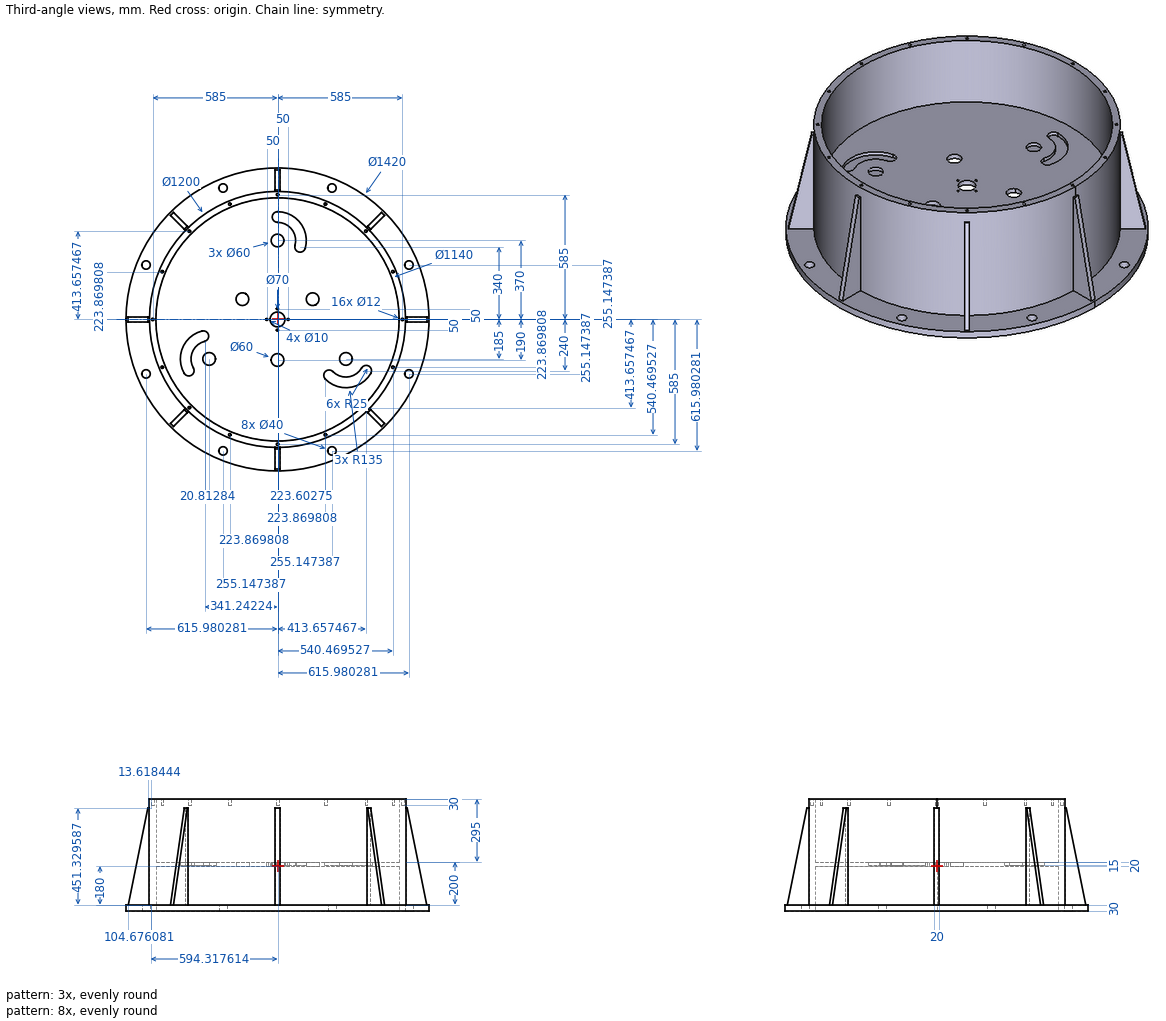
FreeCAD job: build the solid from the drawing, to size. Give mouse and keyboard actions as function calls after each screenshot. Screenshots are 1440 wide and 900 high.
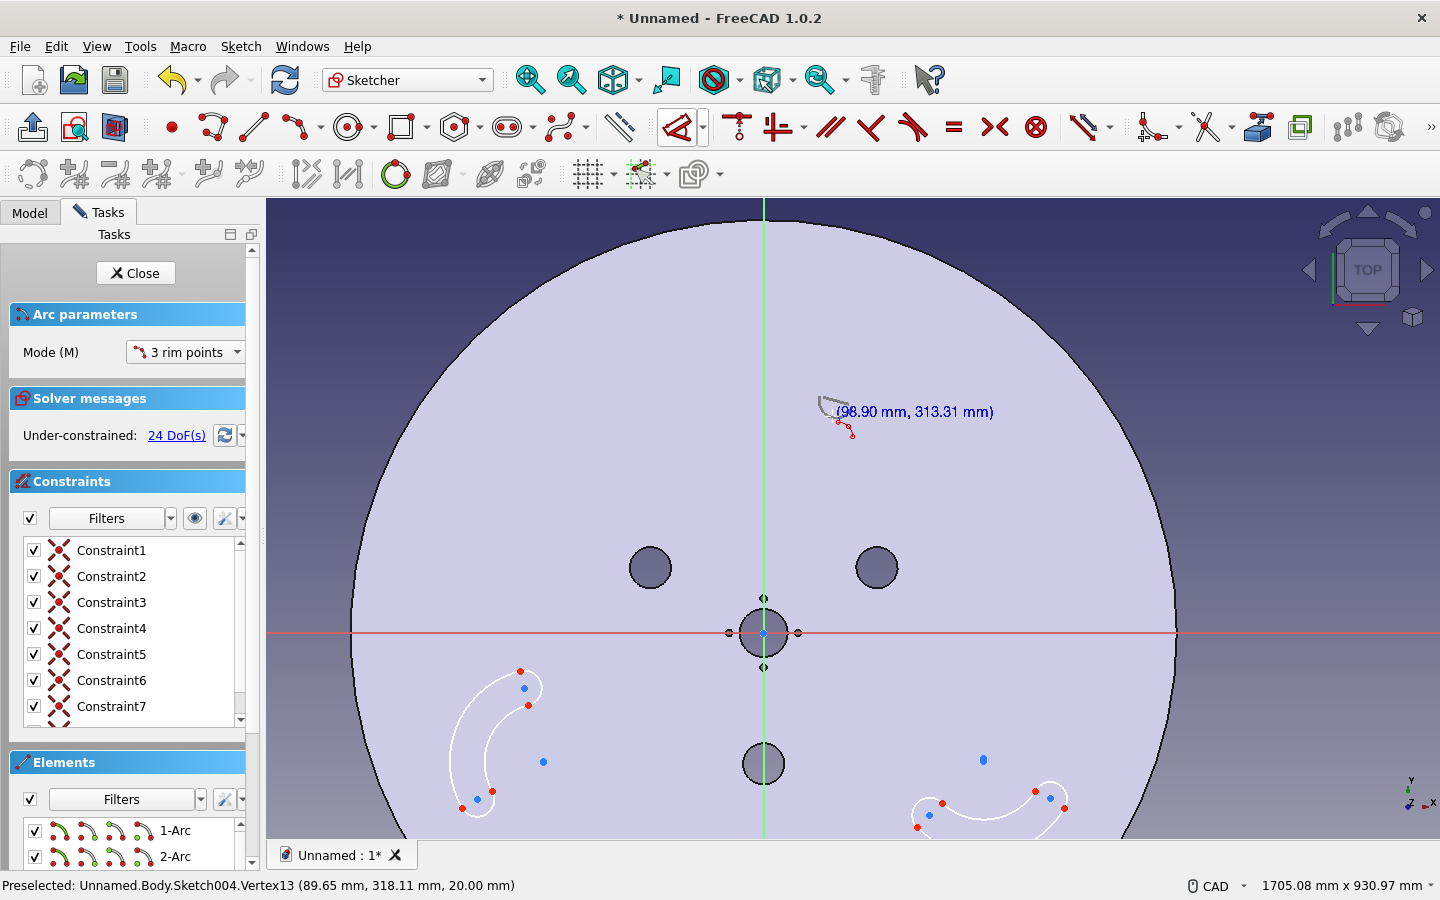
click(832, 416)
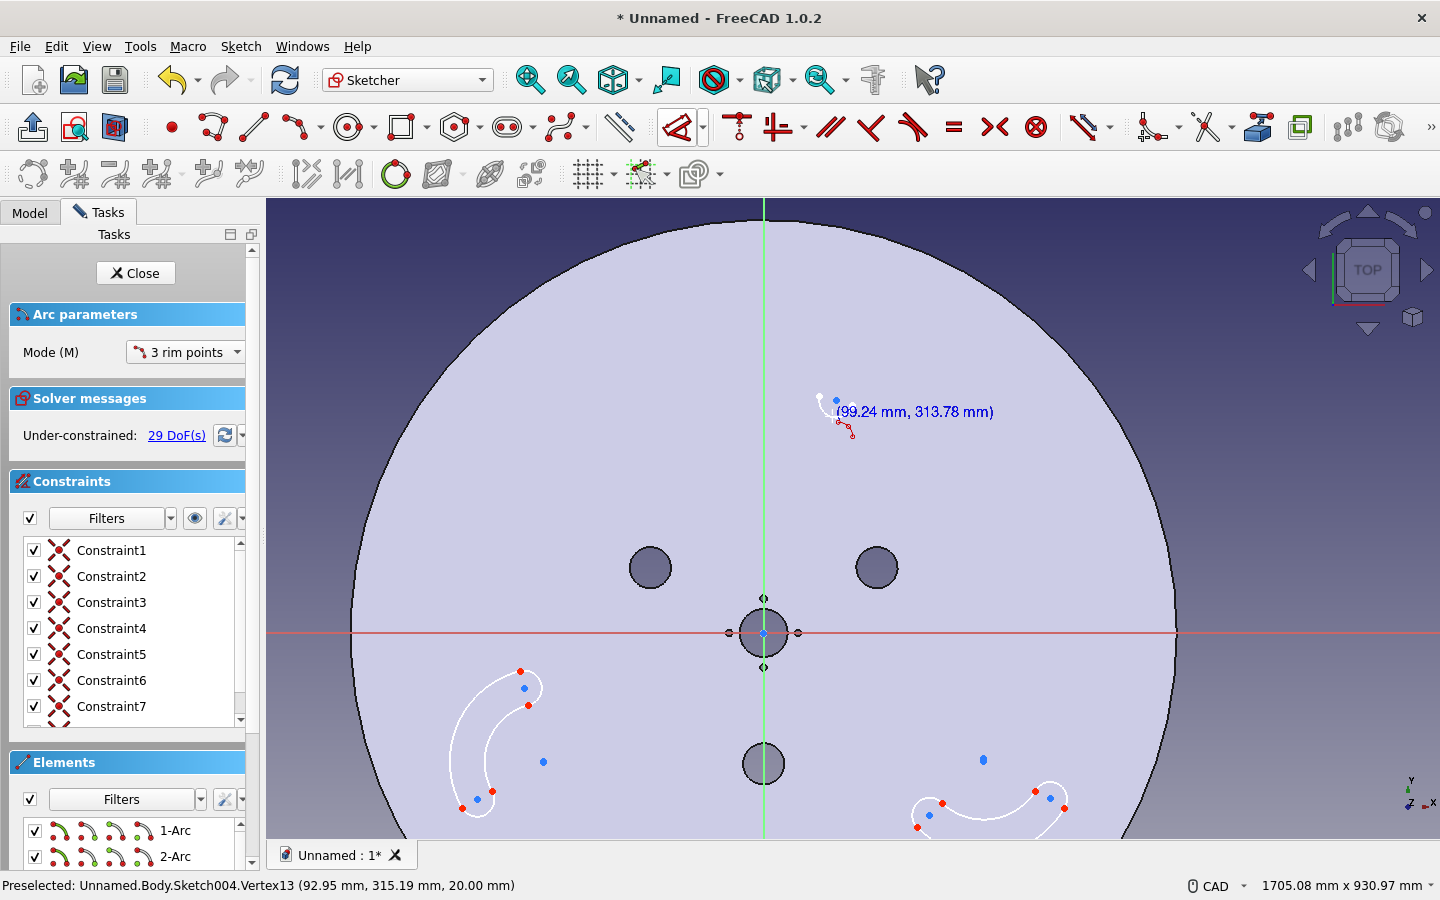
click(853, 405)
click(764, 285)
click(838, 322)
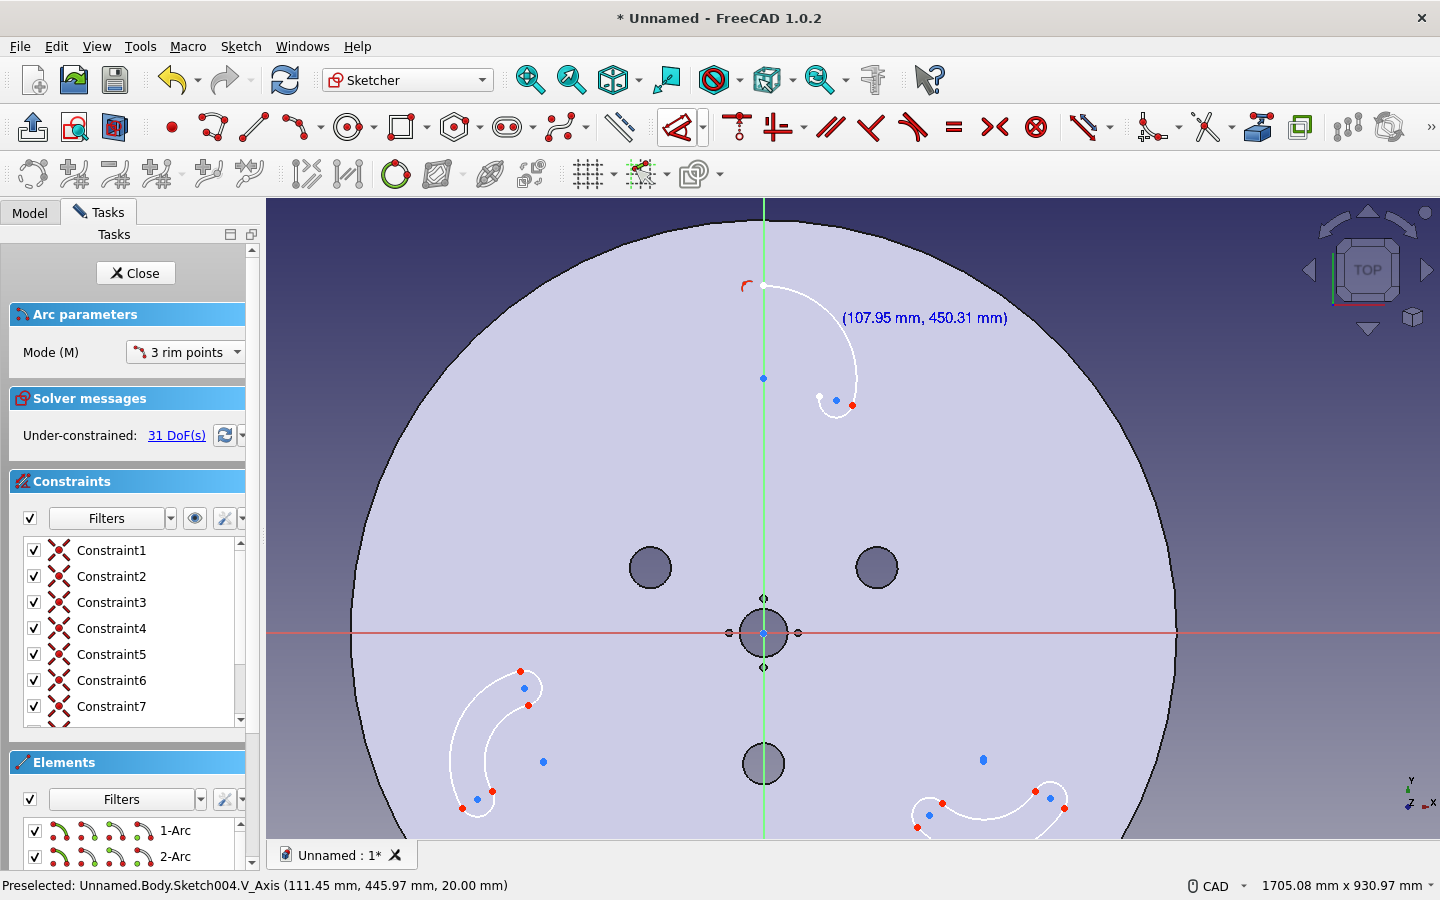
click(764, 286)
click(764, 320)
click(746, 303)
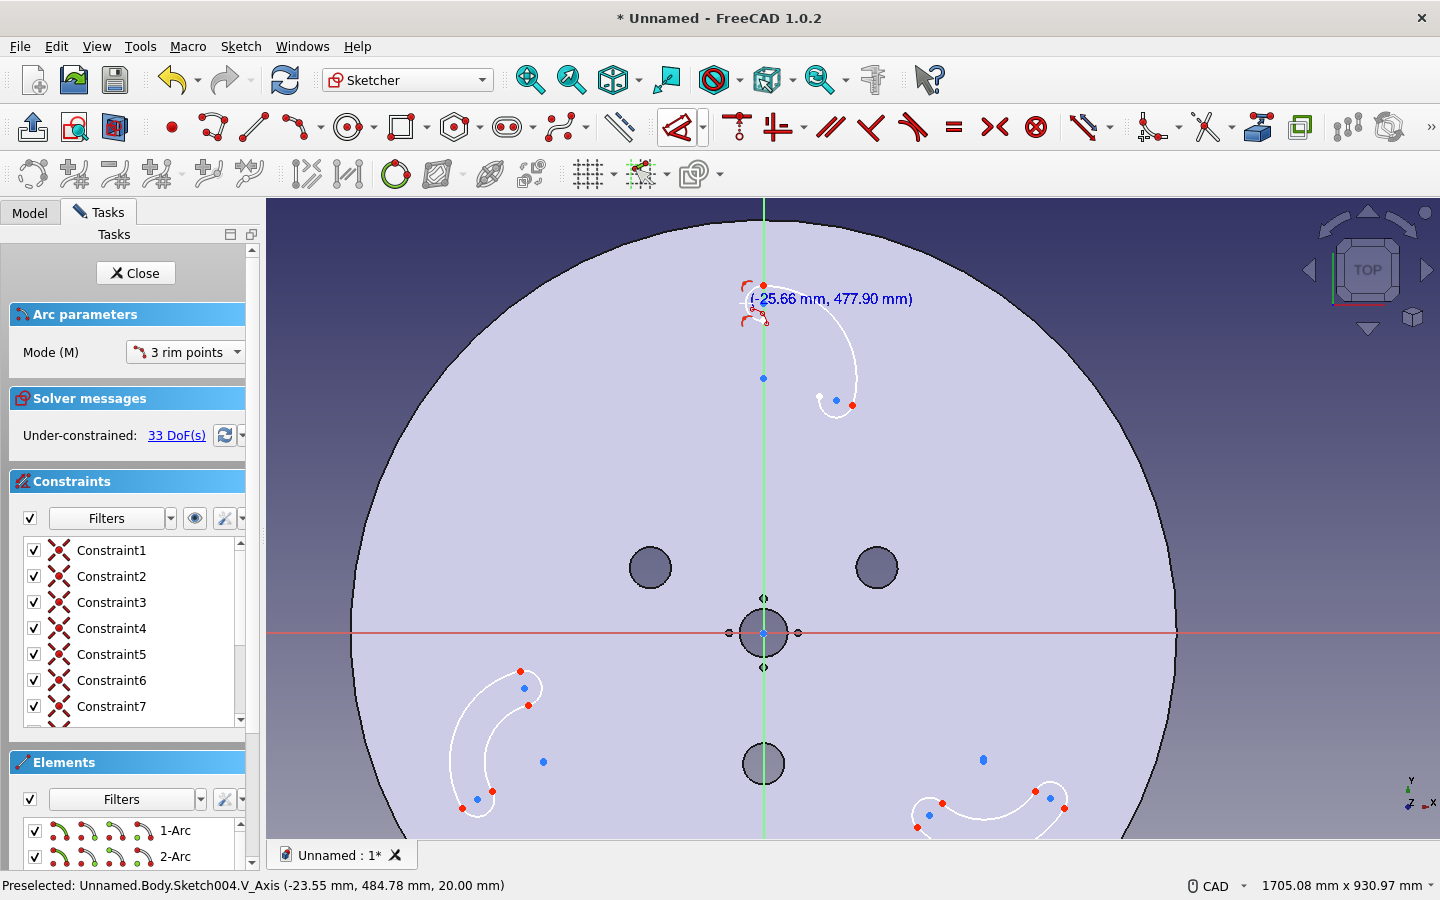
click(764, 321)
click(820, 396)
click(810, 343)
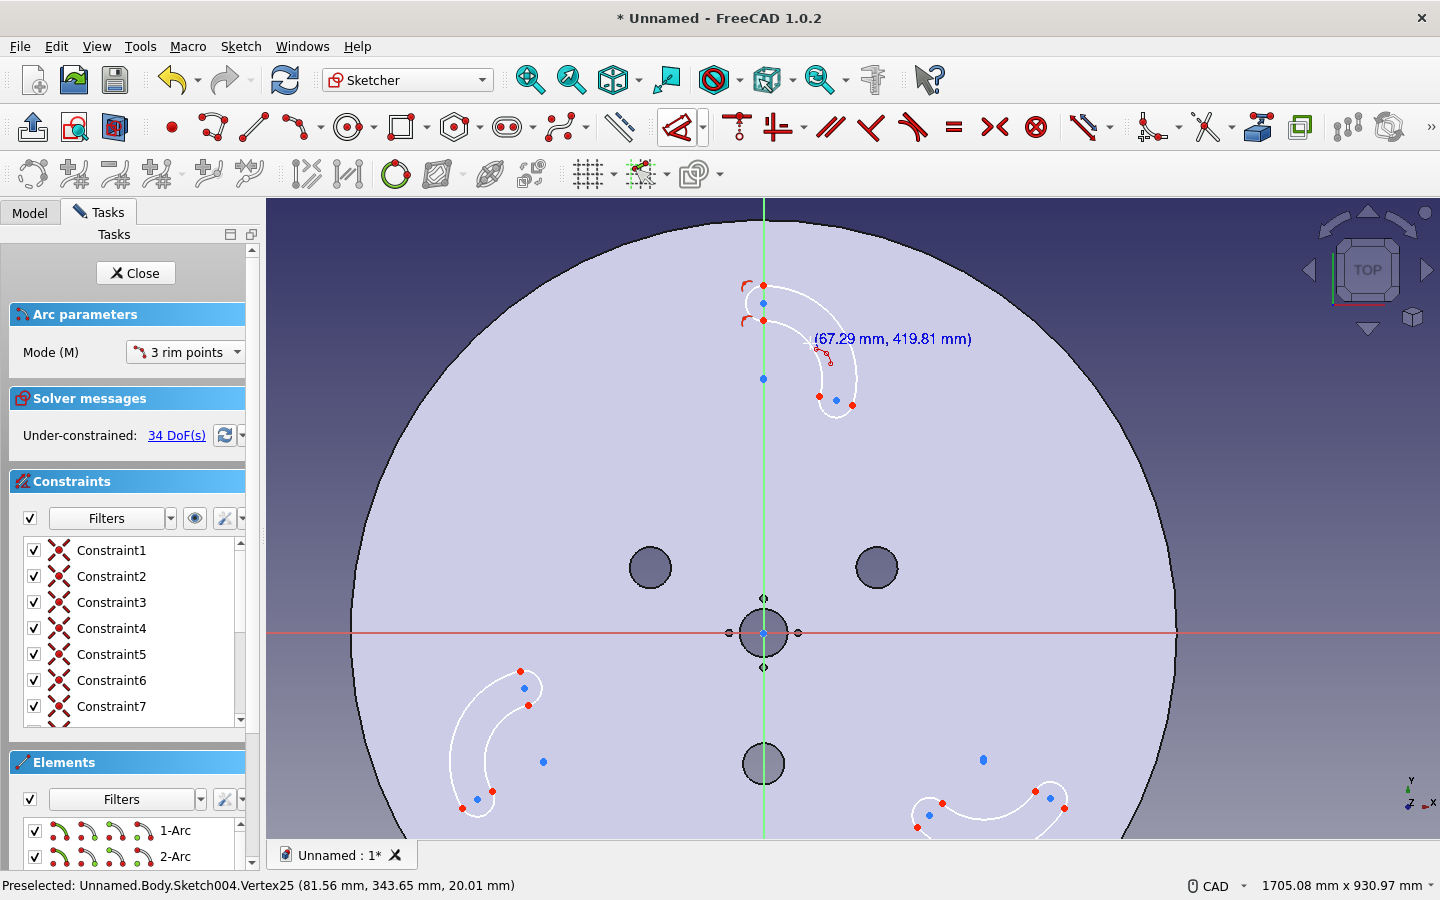
key(g)
key(c)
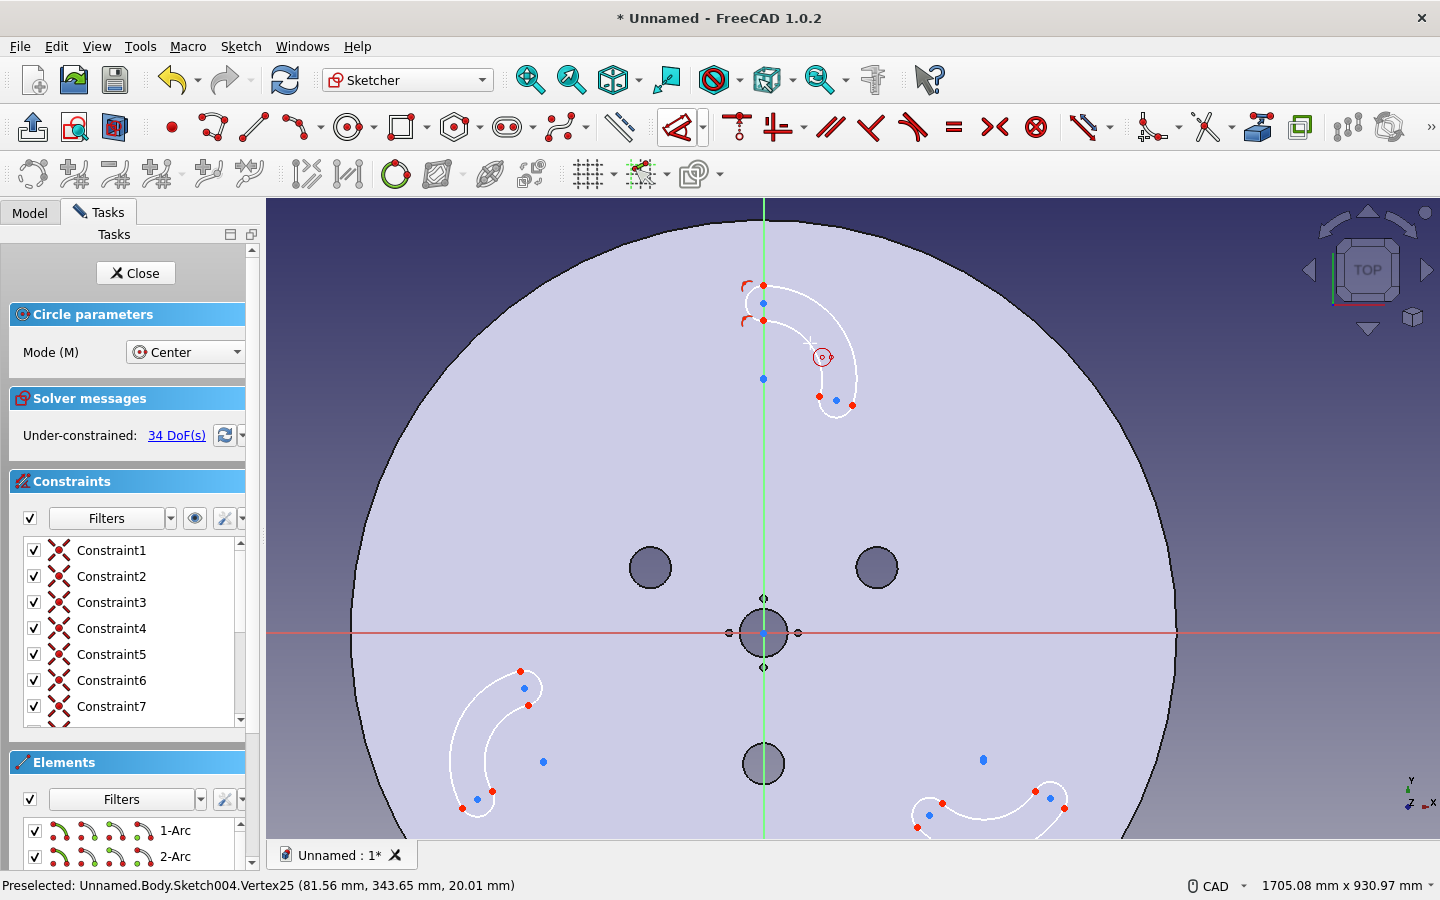
click(764, 378)
move(778, 364)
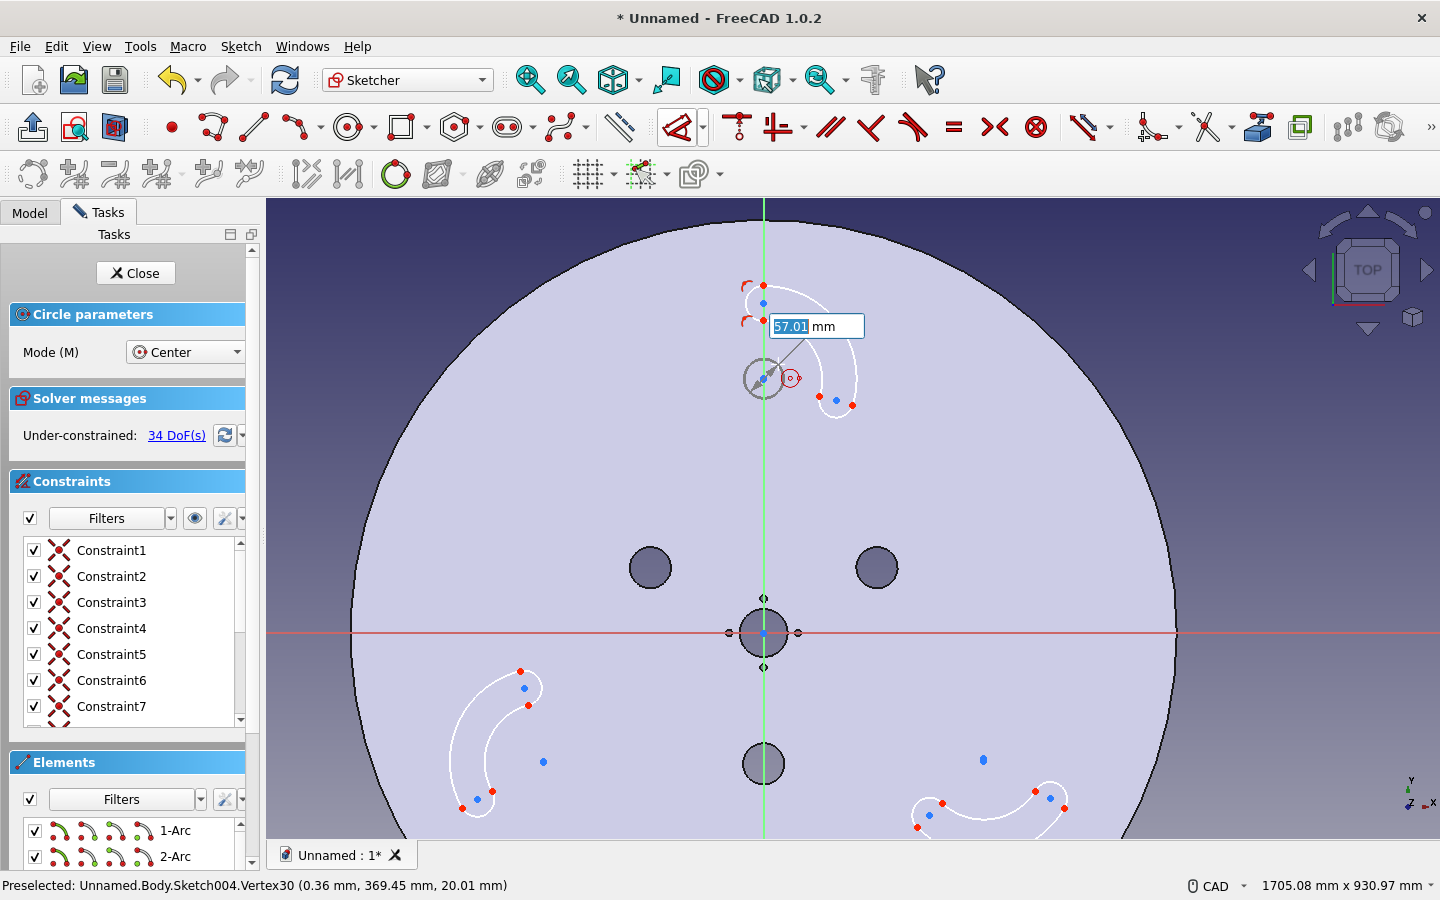
text(60)
key(Return)